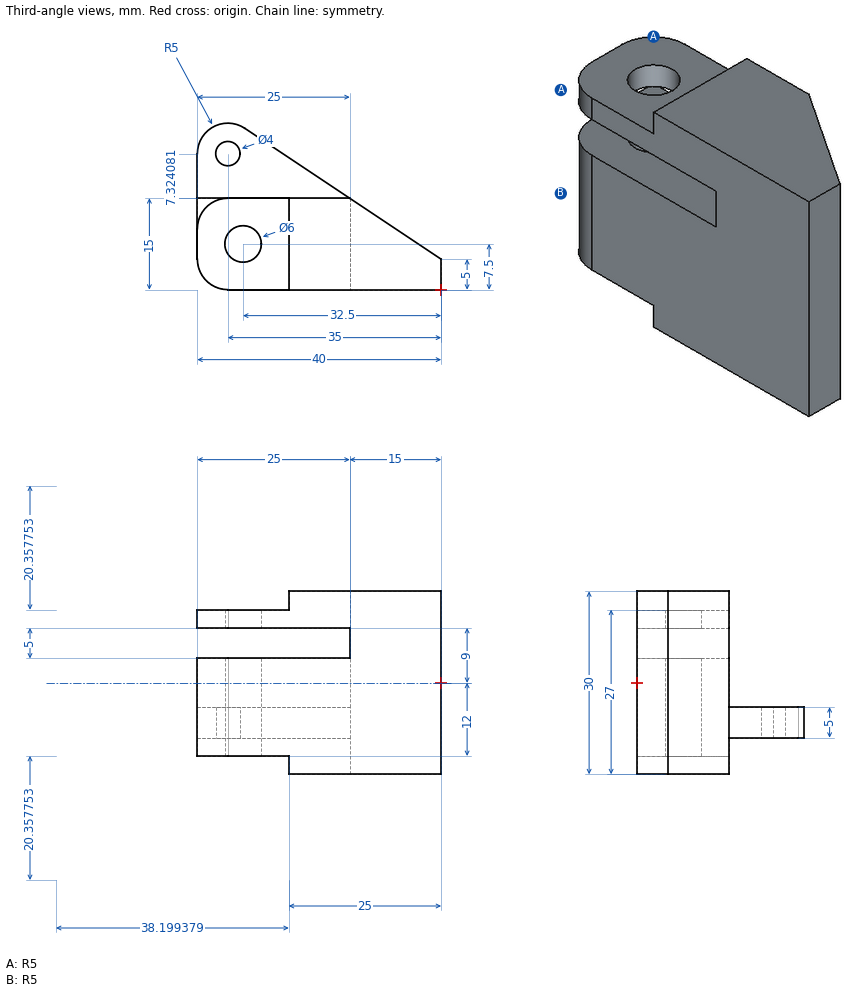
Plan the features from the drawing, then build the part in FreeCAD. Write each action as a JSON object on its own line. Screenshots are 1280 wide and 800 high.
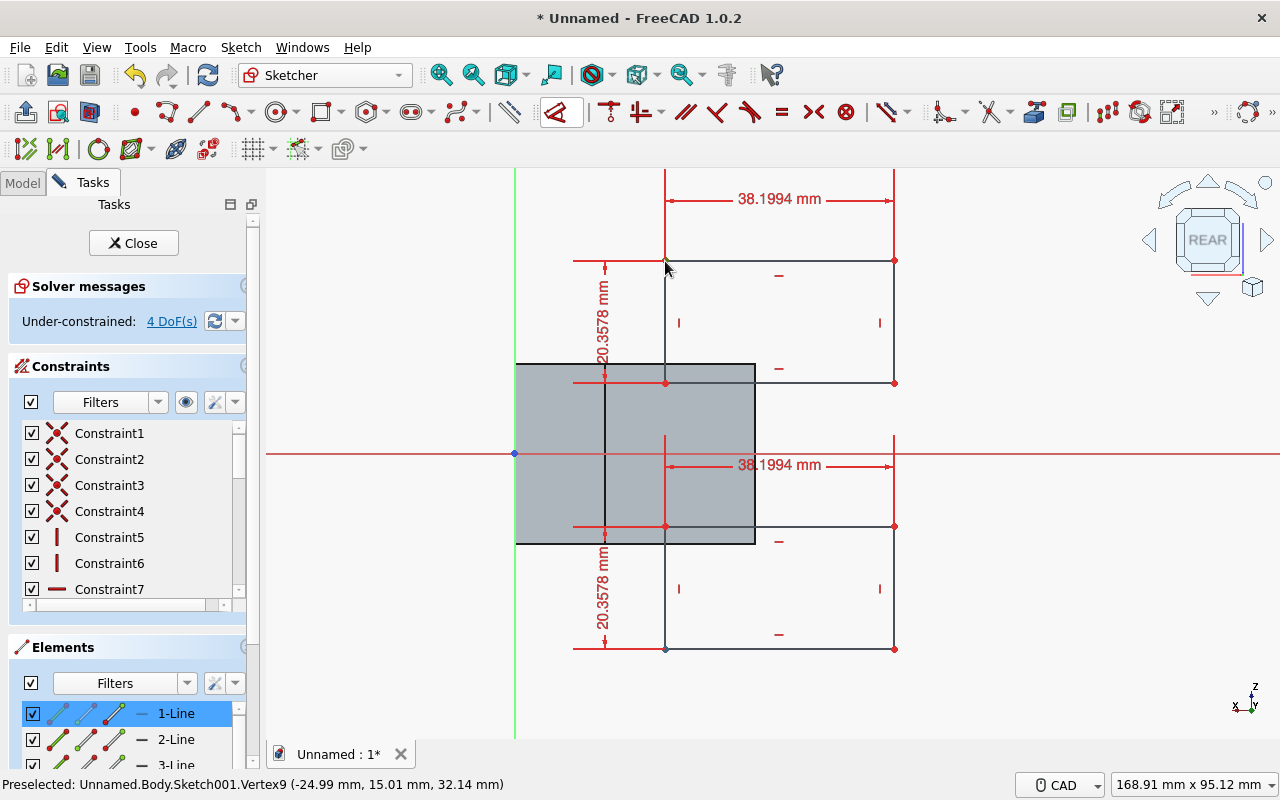
{"action": "left_click", "coordinate": [353, 454]}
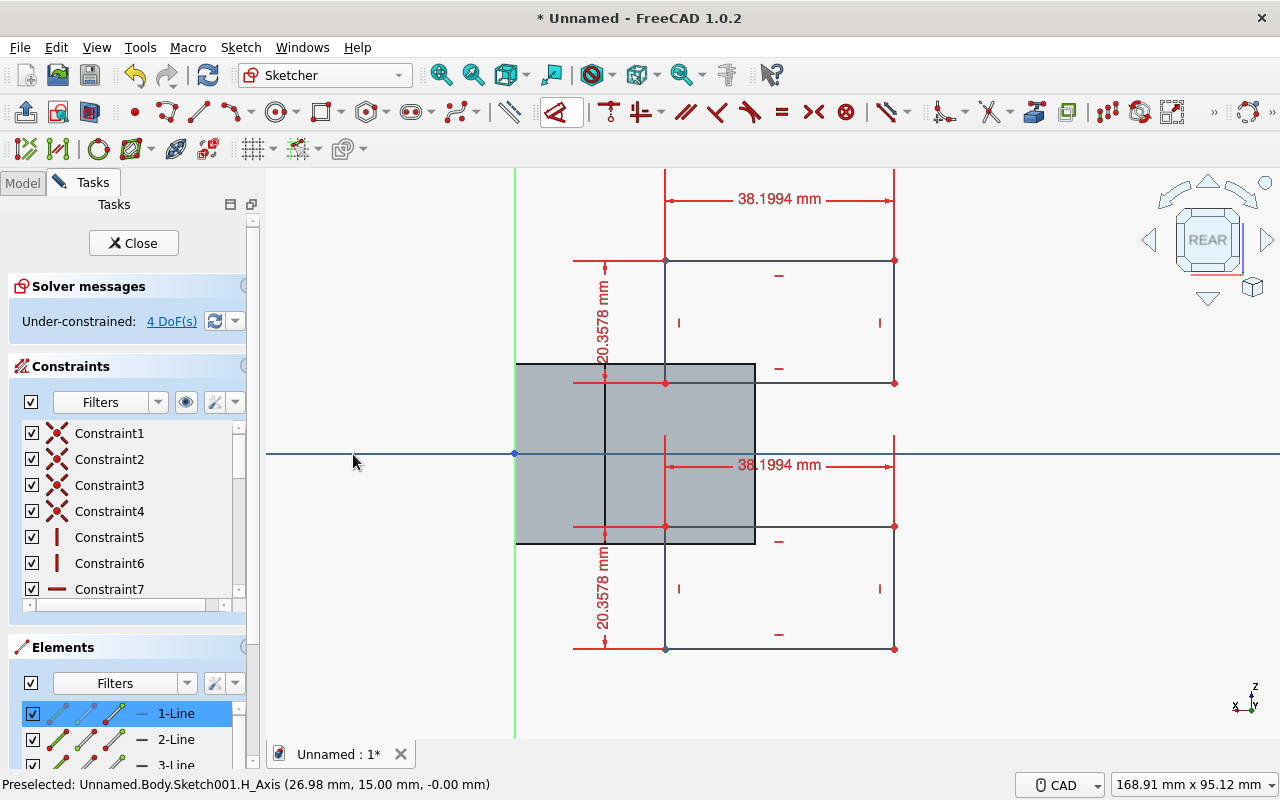
{"action": "key", "text": "s"}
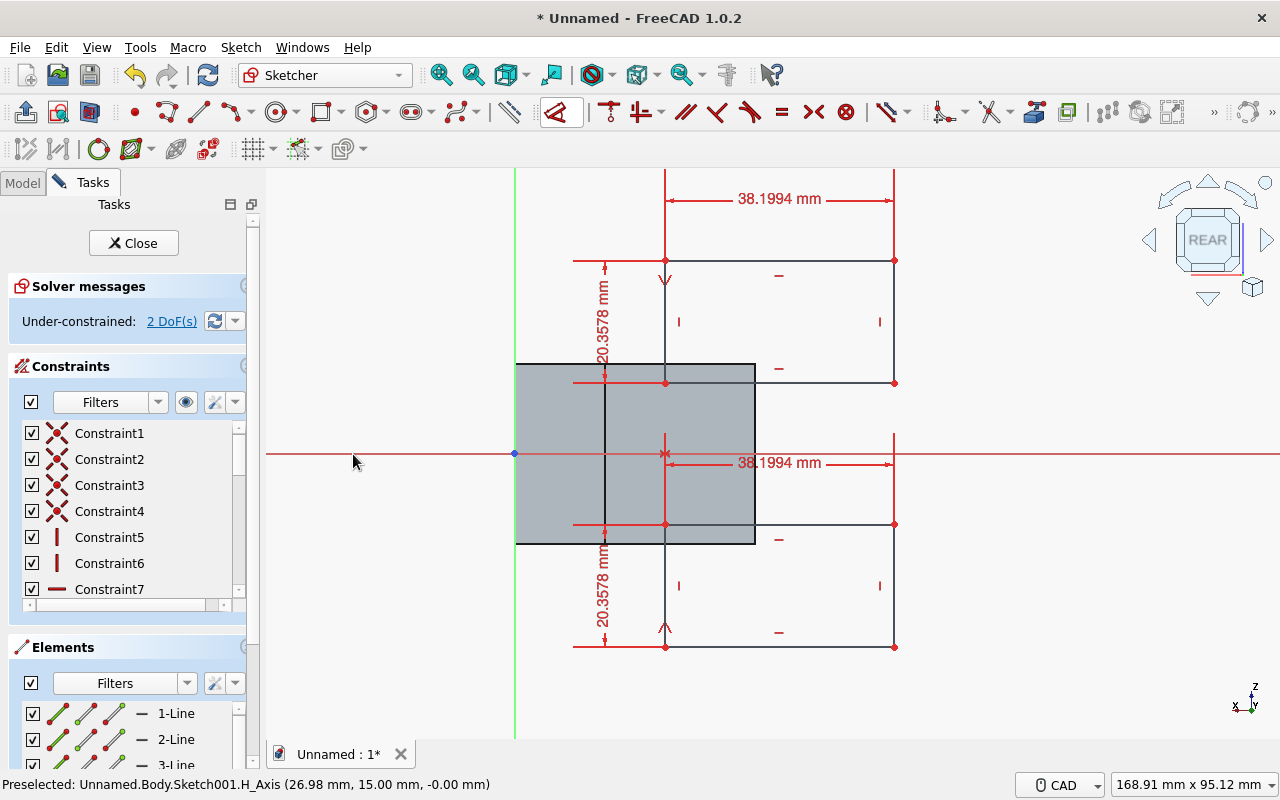
{"action": "left_click", "coordinate": [665, 525]}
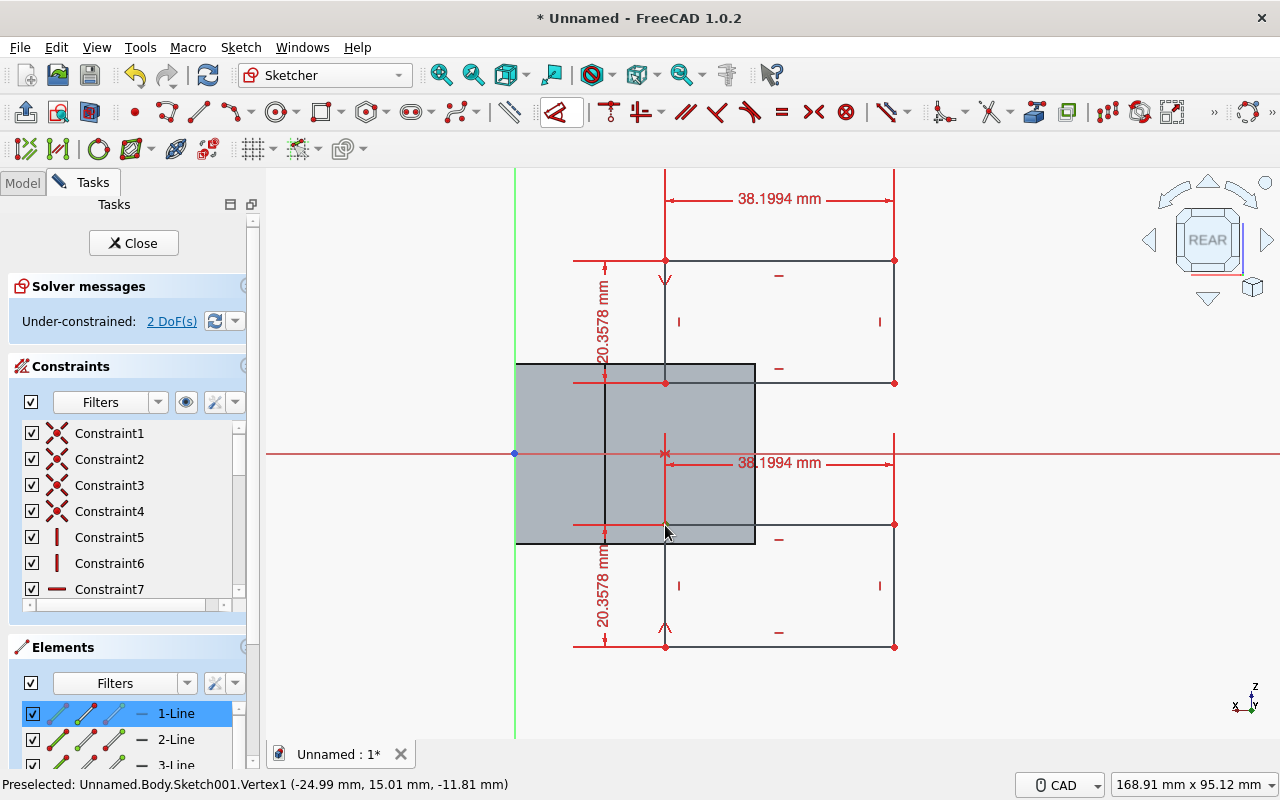
{"action": "key", "text": "l"}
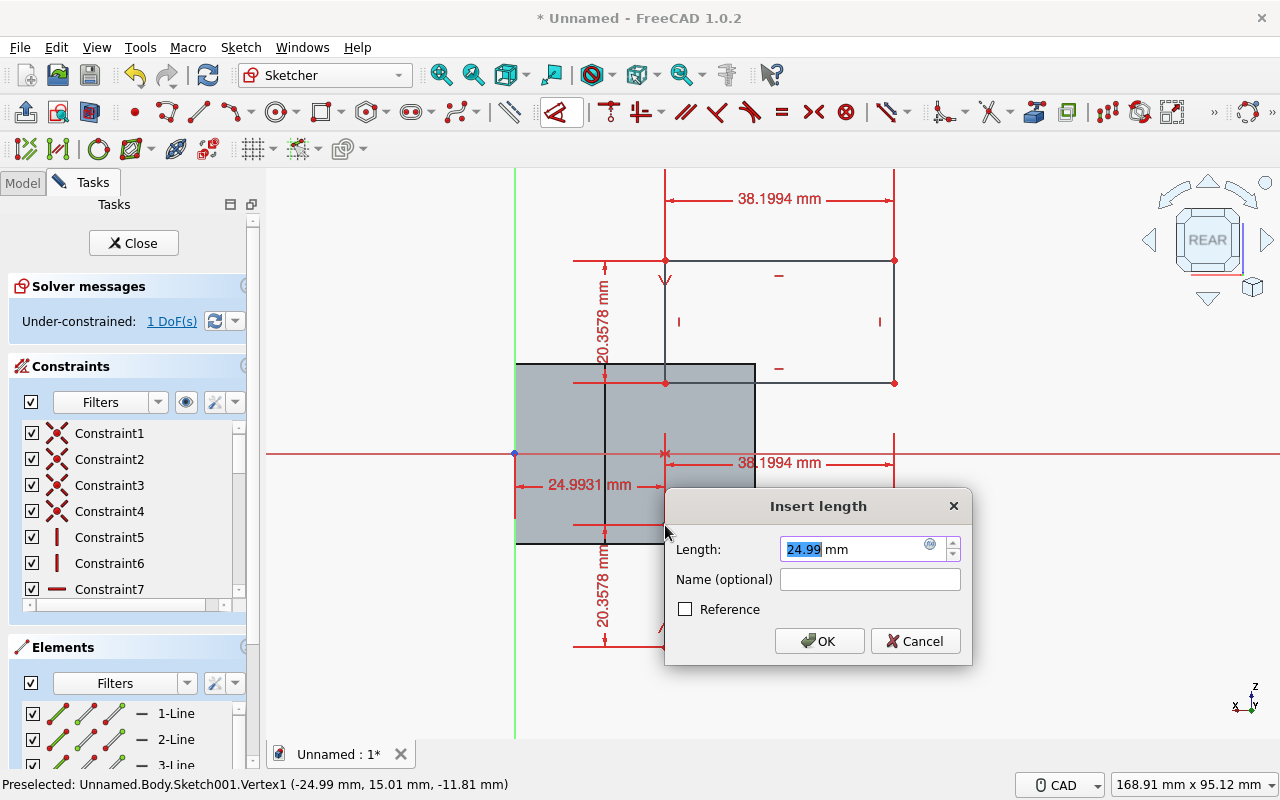
{"action": "type", "text": "25"}
{"action": "key", "text": "Return"}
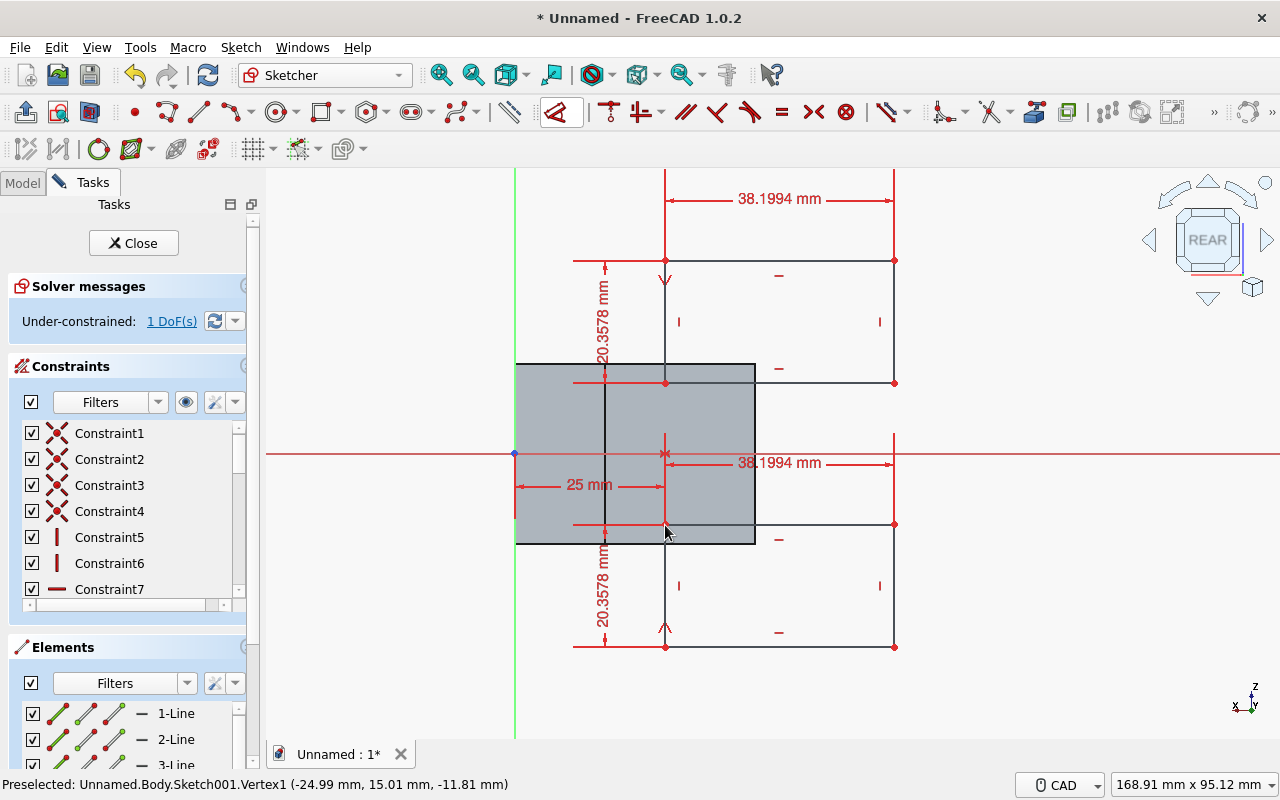
{"action": "left_click", "coordinate": [665, 525]}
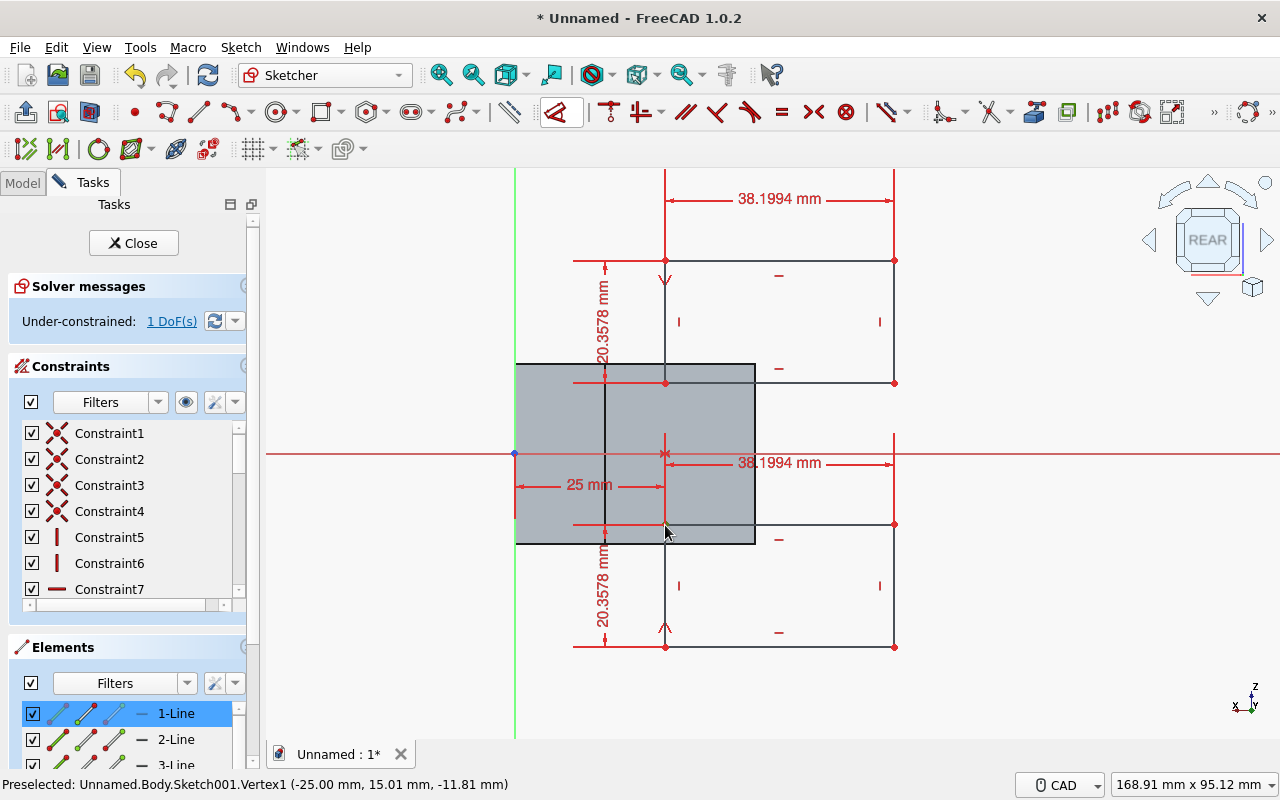
{"action": "key", "text": "i"}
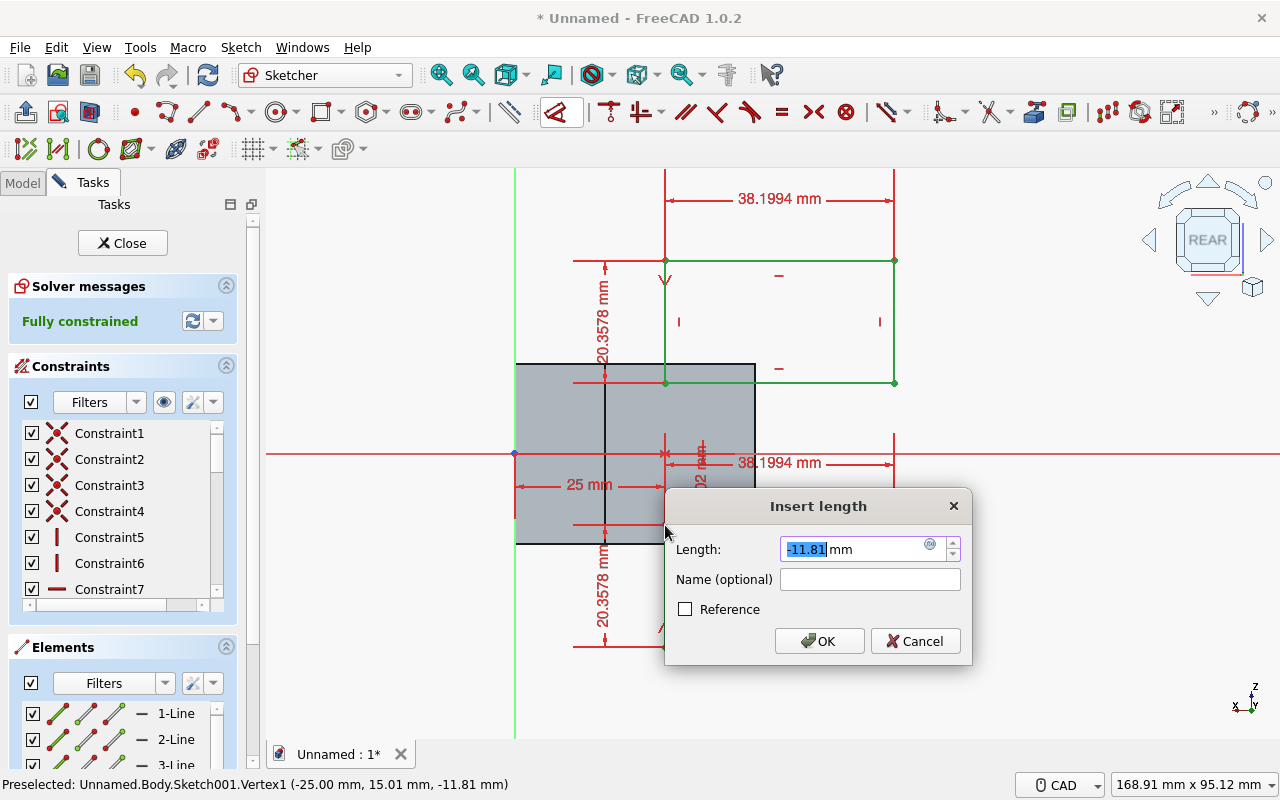
{"action": "type", "text": "-12"}
{"action": "key", "text": "Return"}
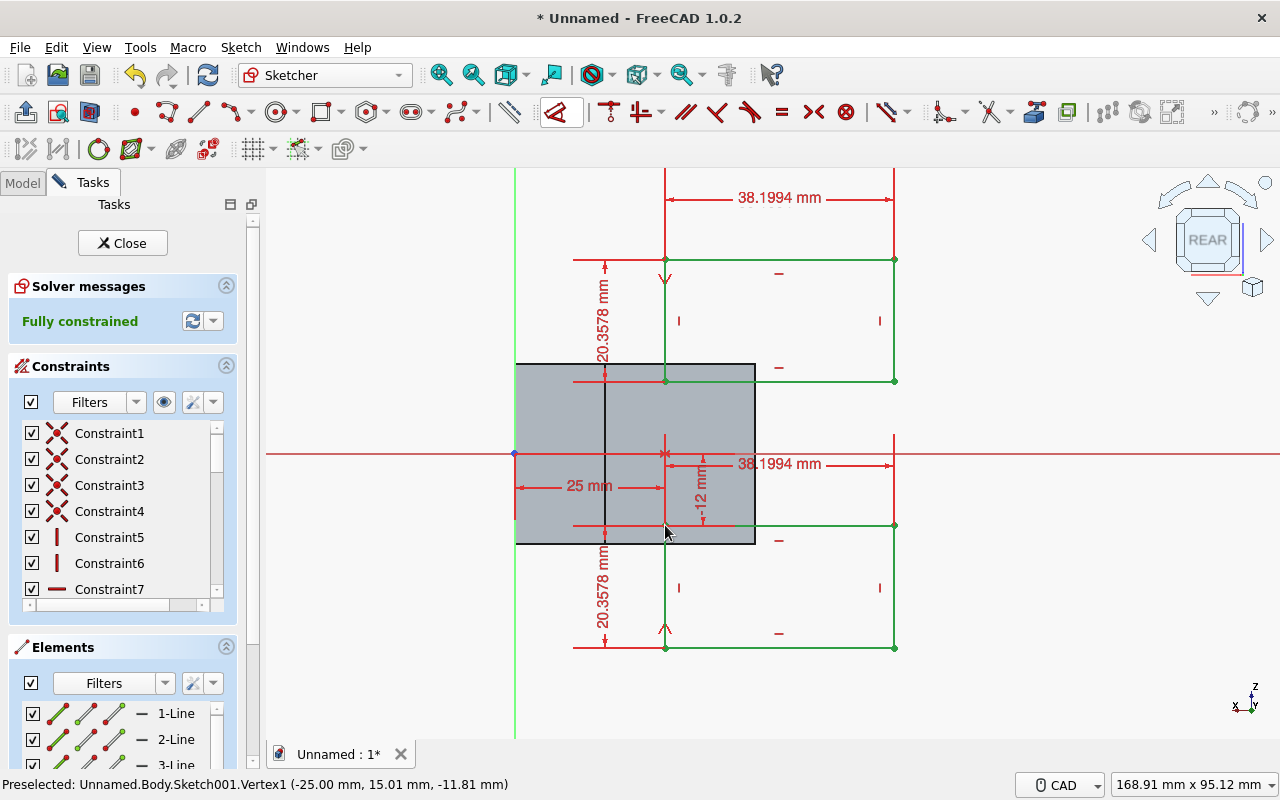
{"action": "left_click", "coordinate": [123, 243]}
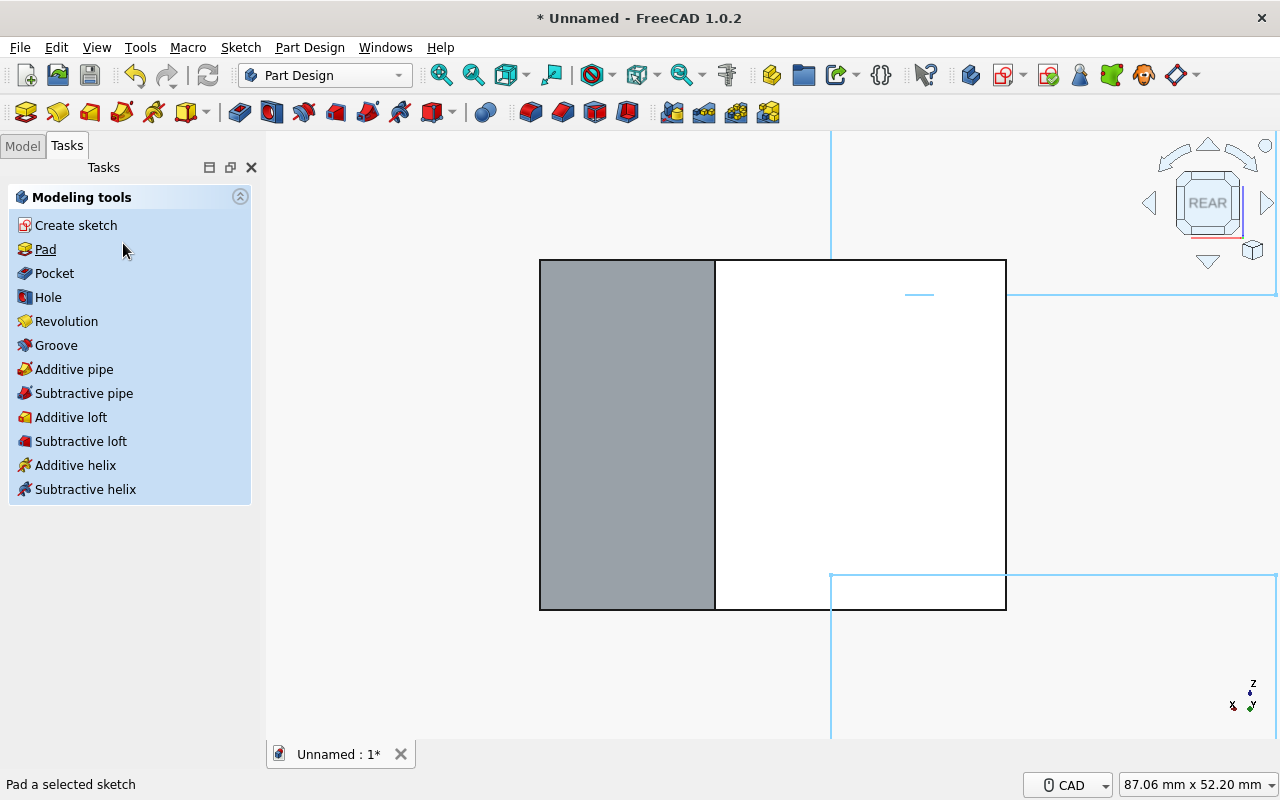
{"action": "left_click", "coordinate": [240, 112]}